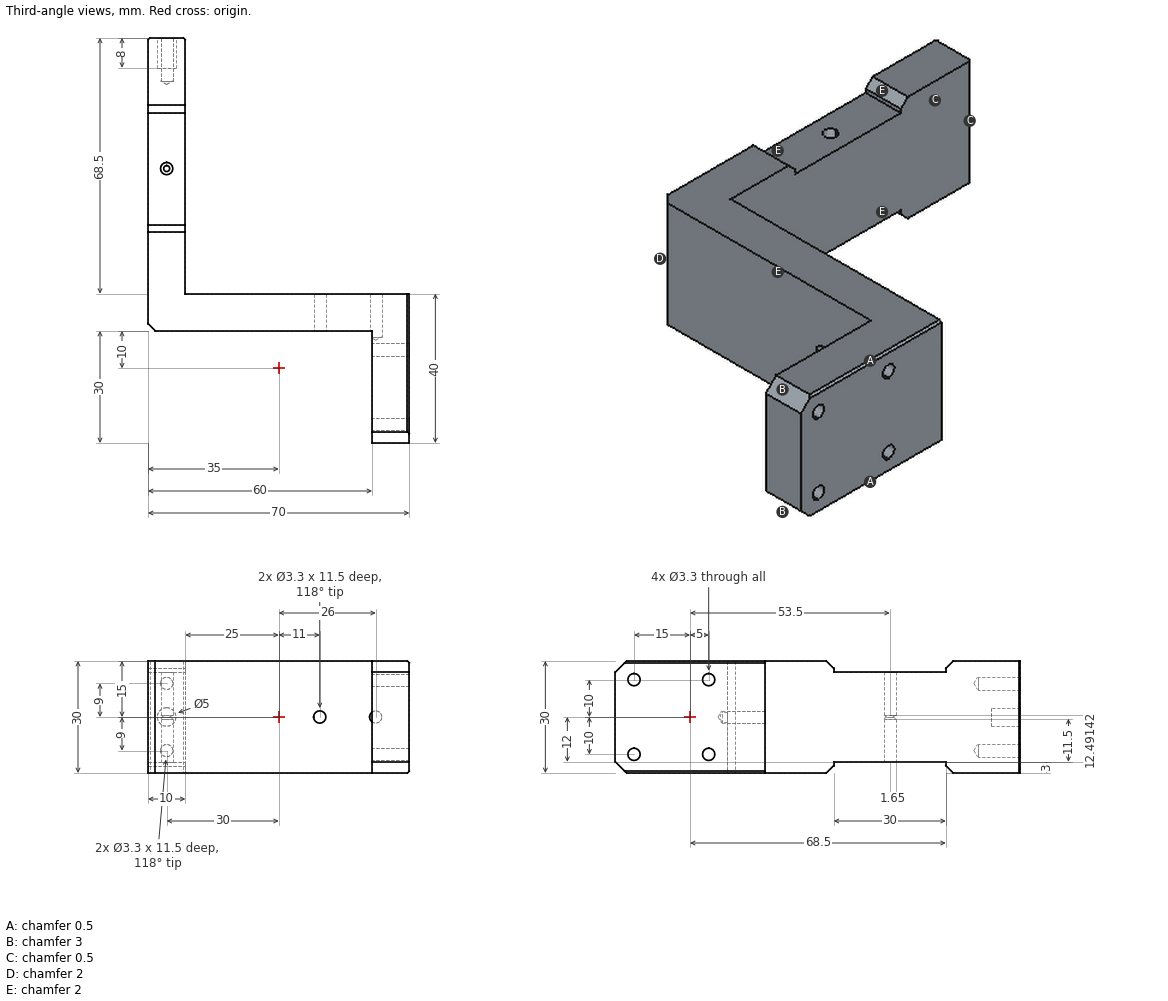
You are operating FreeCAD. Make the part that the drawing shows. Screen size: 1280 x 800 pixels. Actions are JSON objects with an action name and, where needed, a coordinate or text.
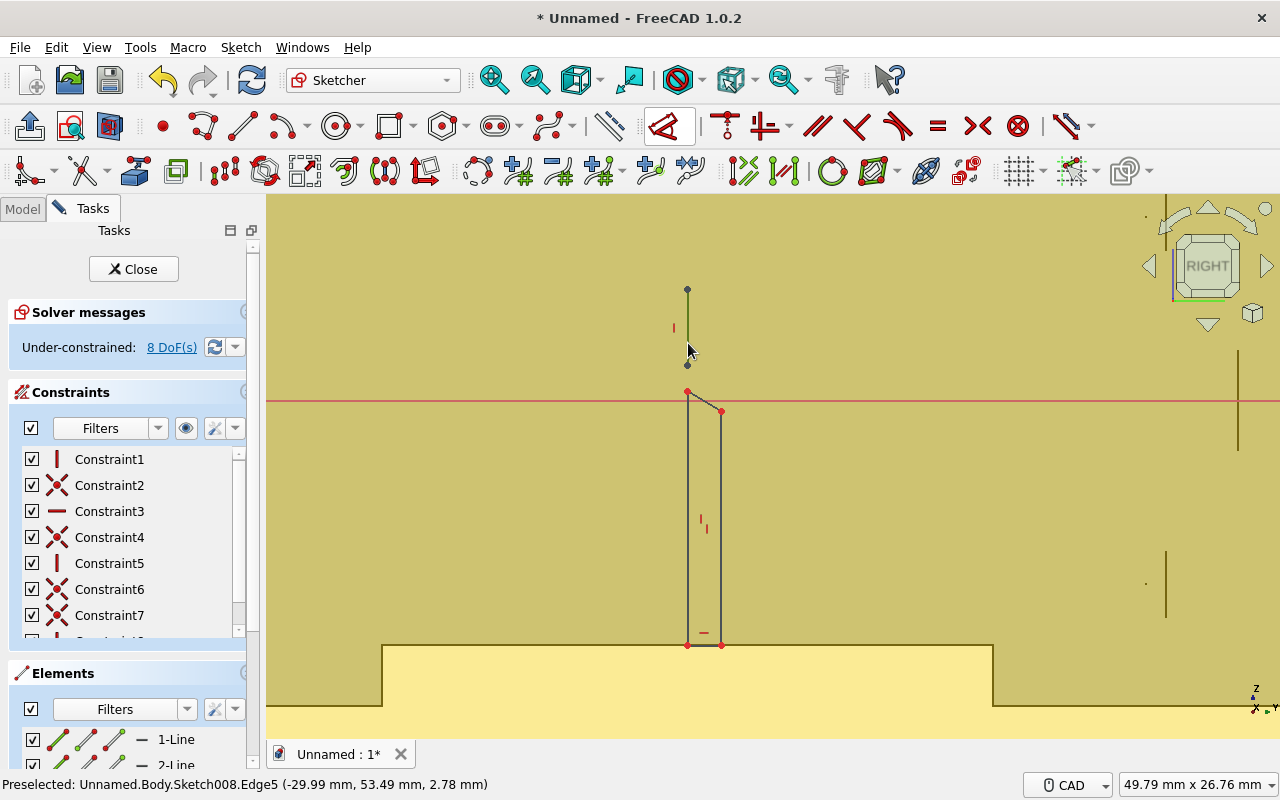
{"action": "left_click", "coordinate": [610, 126]}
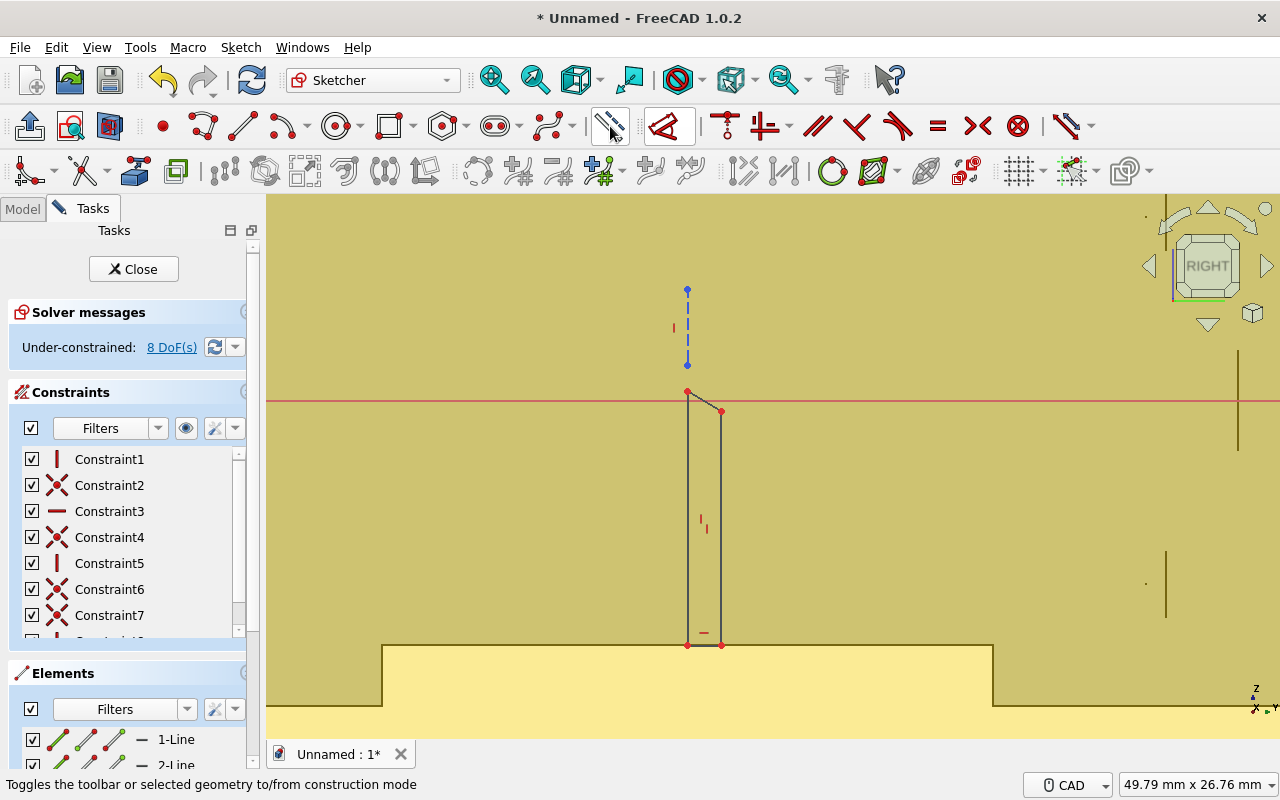
{"action": "left_click", "coordinate": [688, 646]}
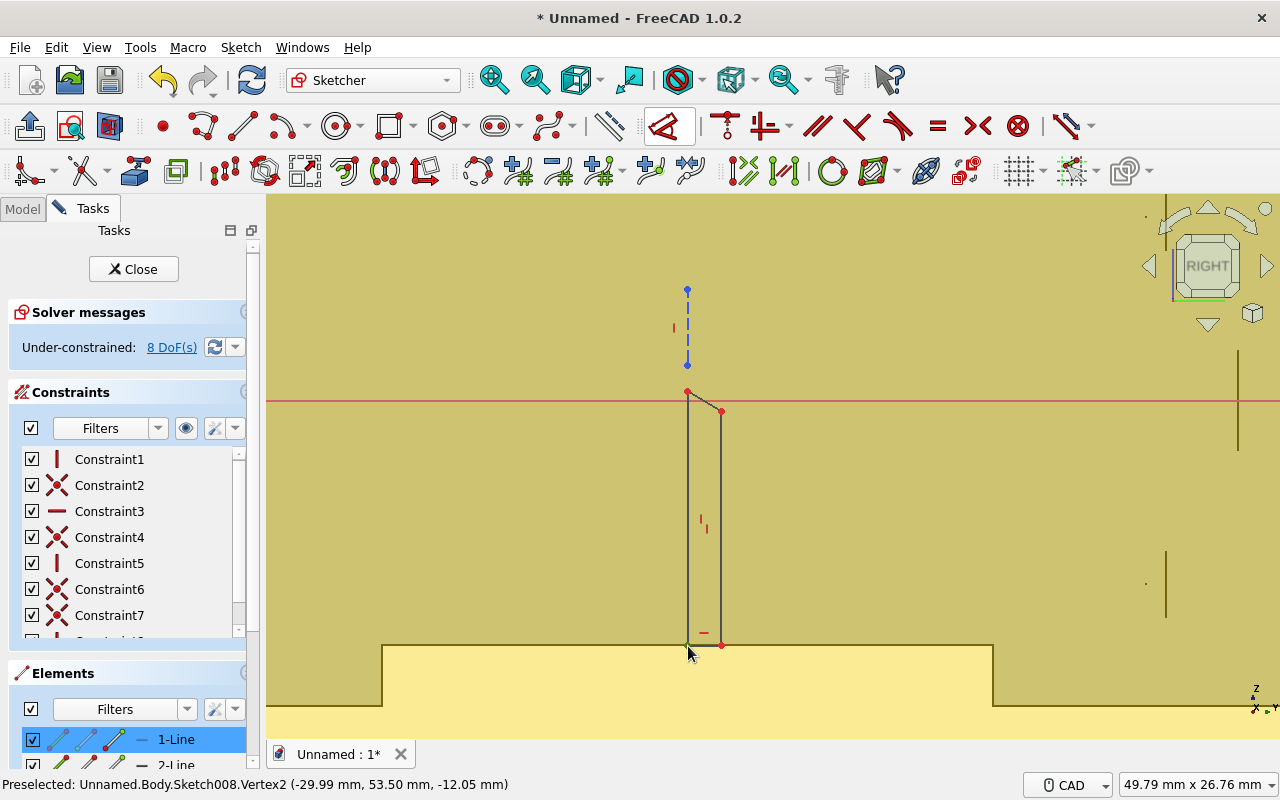
{"action": "key", "text": "i"}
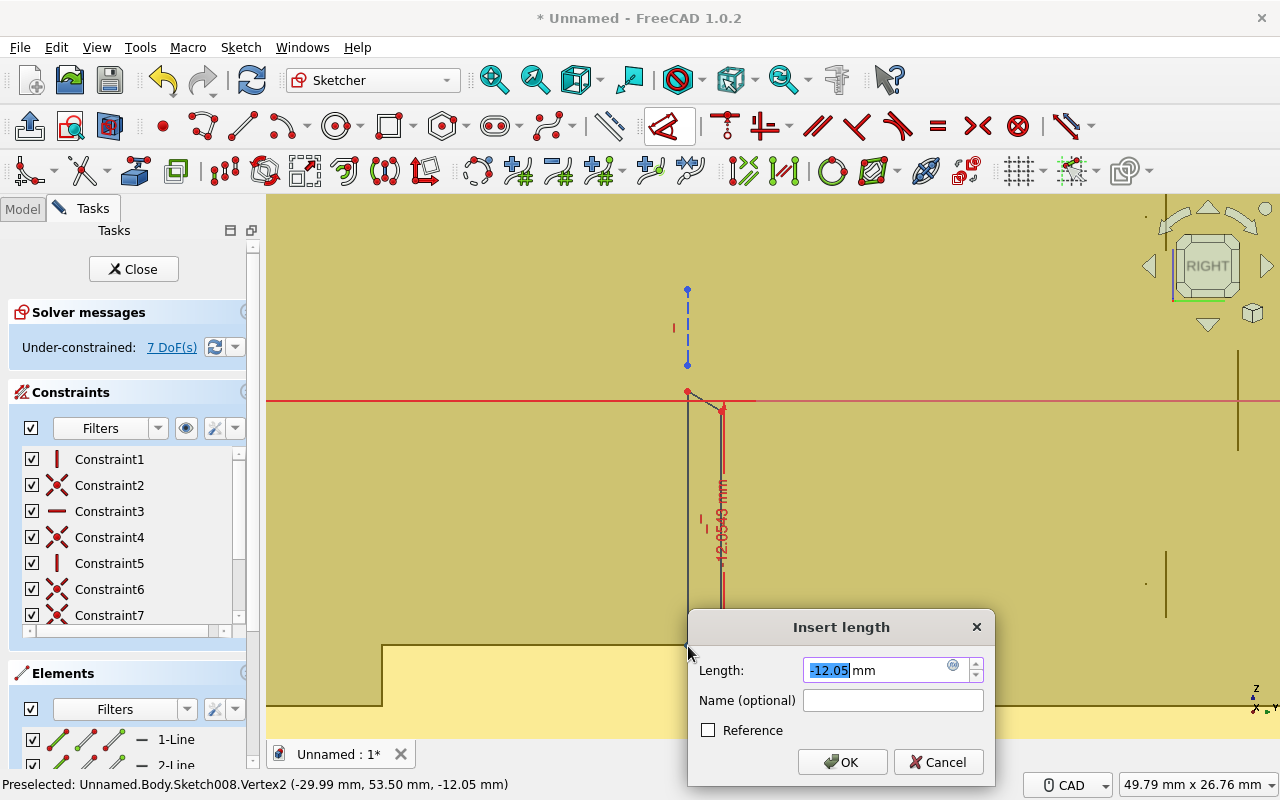
{"action": "type", "text": "-12"}
{"action": "key", "text": "Return"}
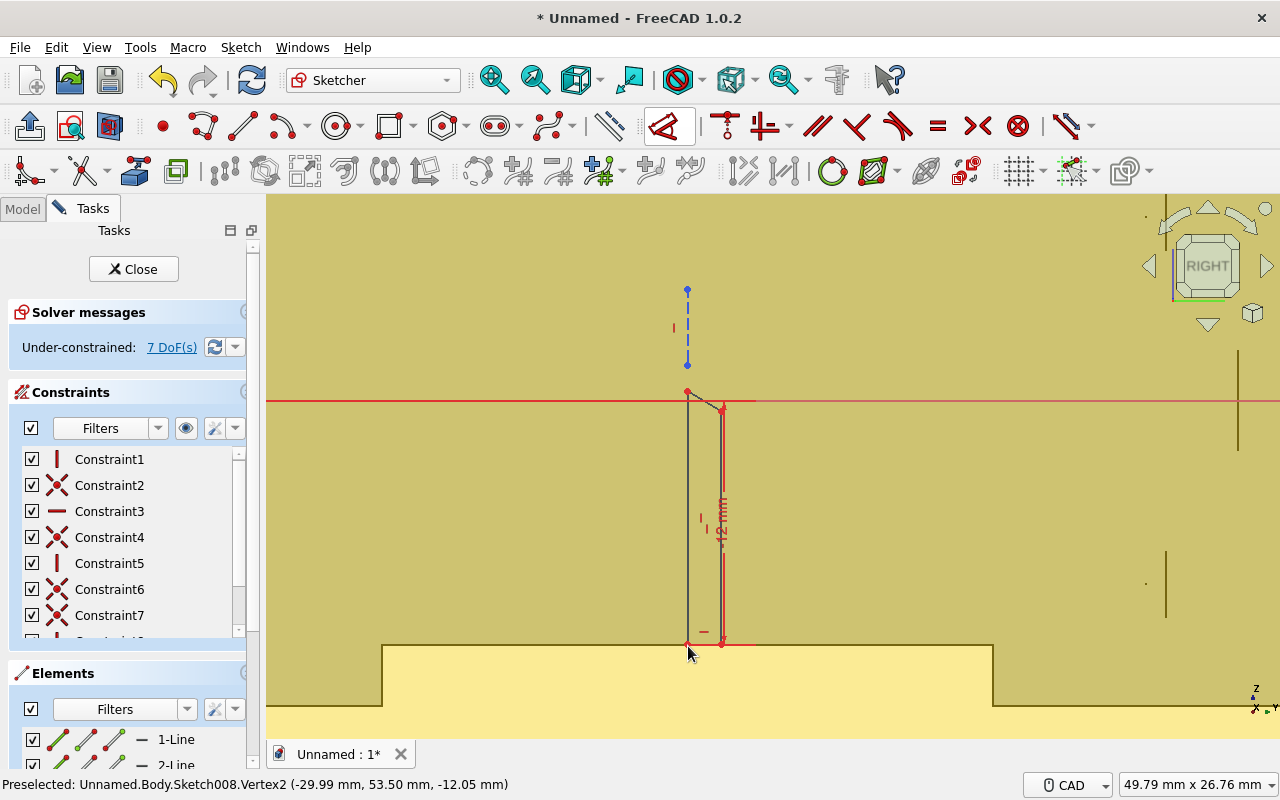
{"action": "scroll", "coordinate": [698, 645], "scroll_direction": "up", "scroll_amount": 2}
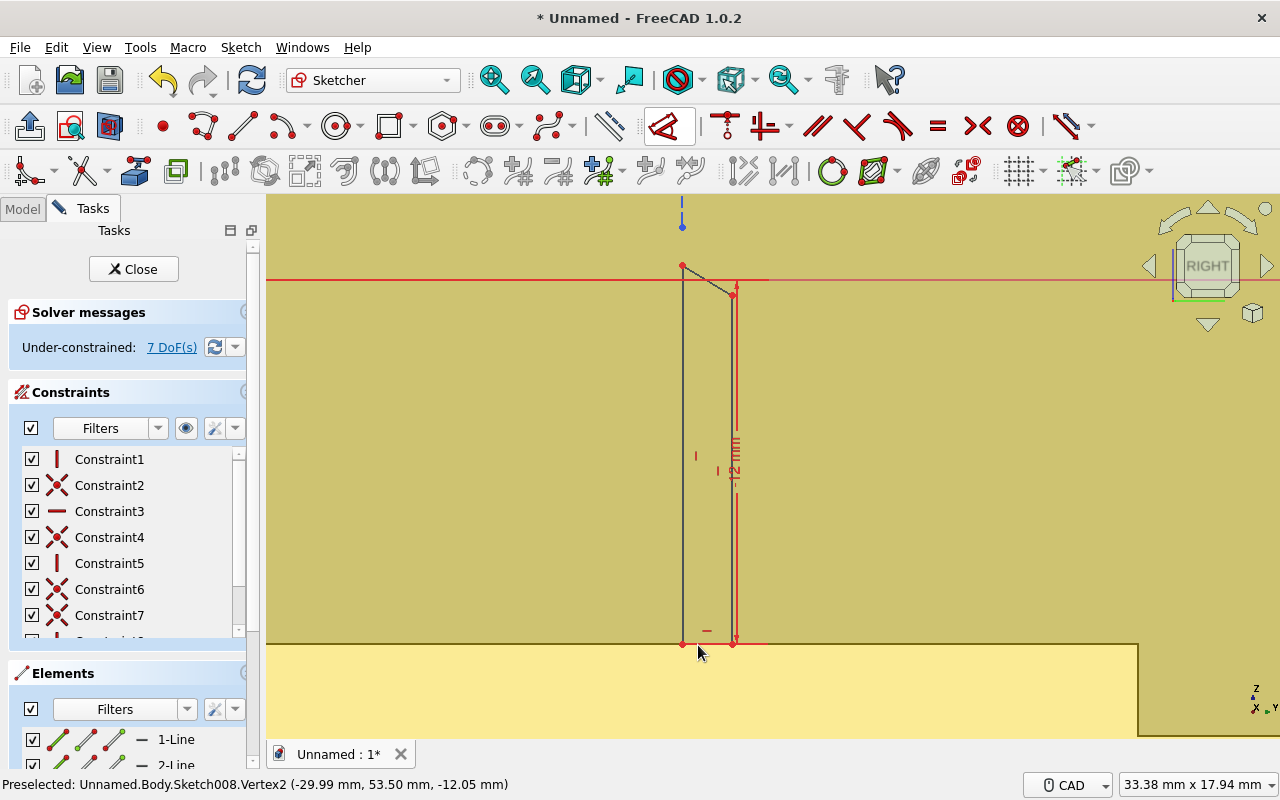
{"action": "left_click", "coordinate": [697, 644]}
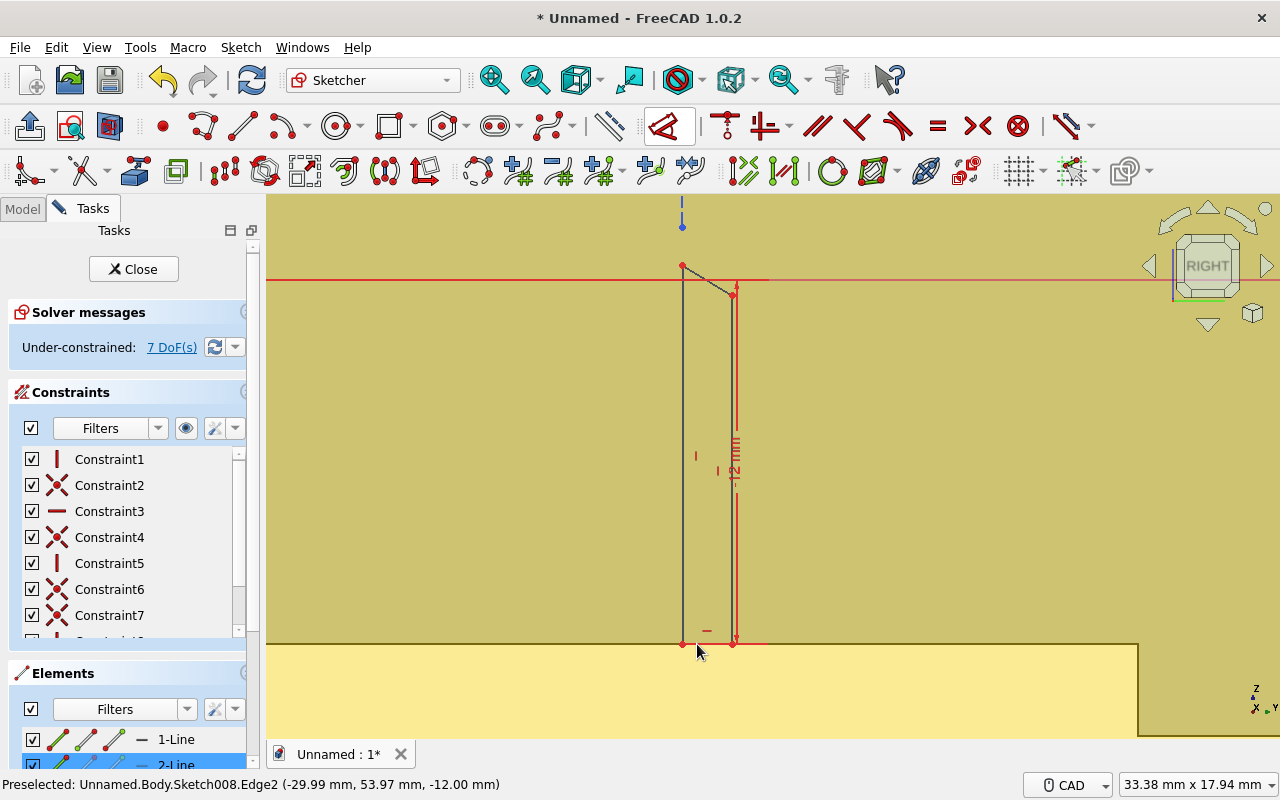
{"action": "left_click", "coordinate": [690, 126]}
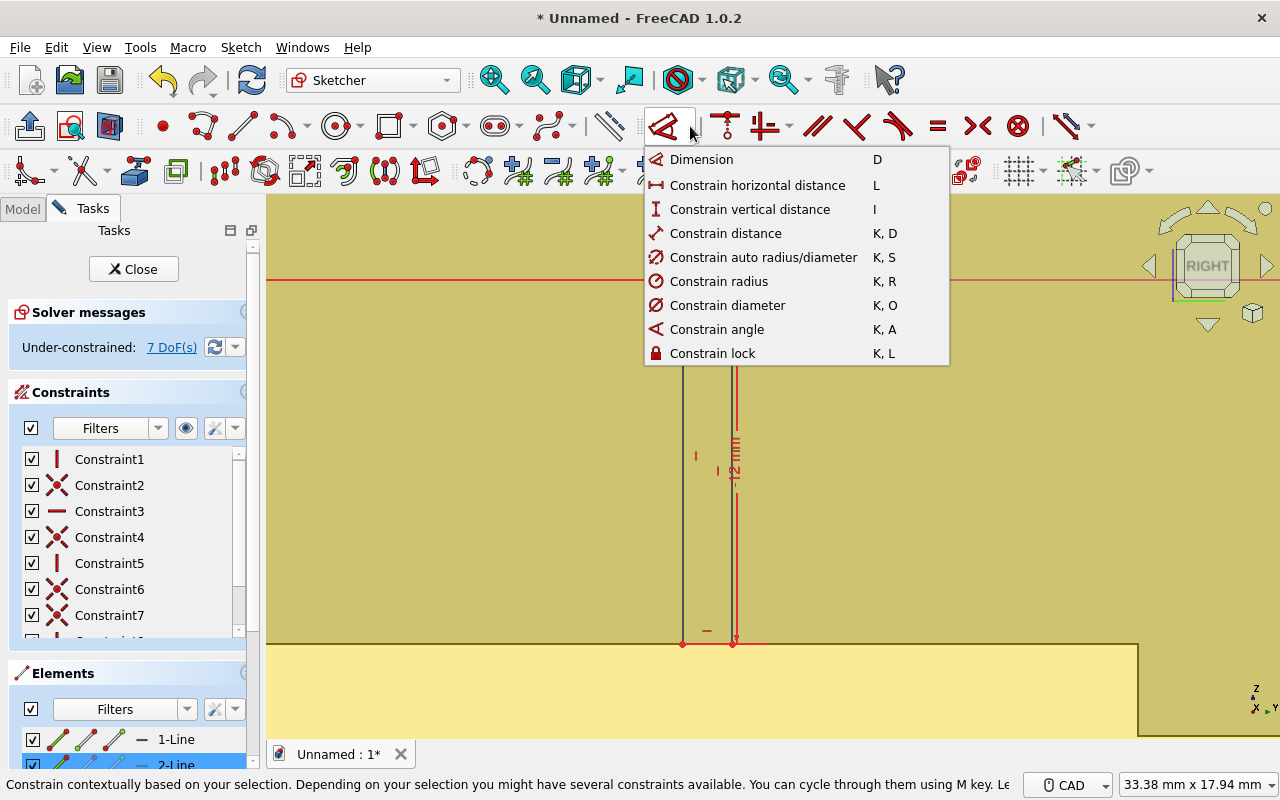
{"action": "left_click", "coordinate": [797, 185]}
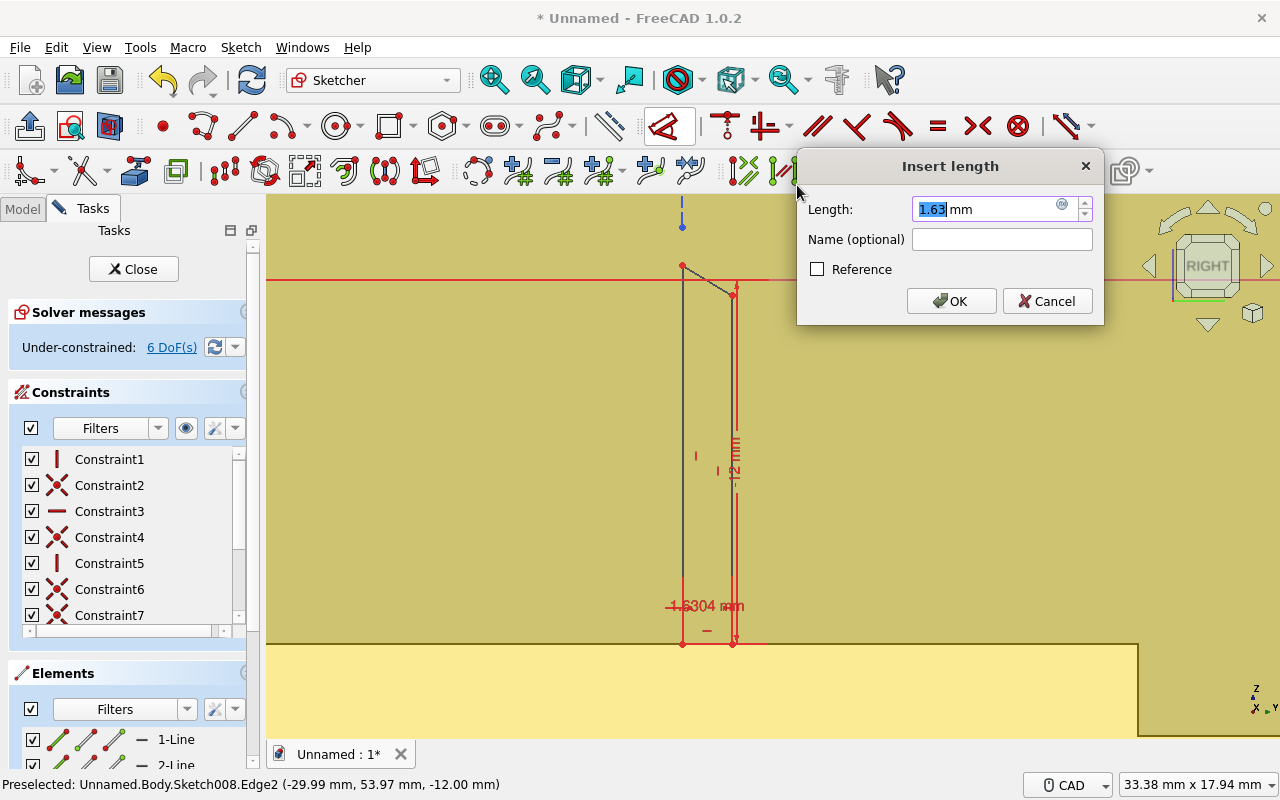
{"action": "type", "text": "1.65"}
{"action": "key", "text": "Return"}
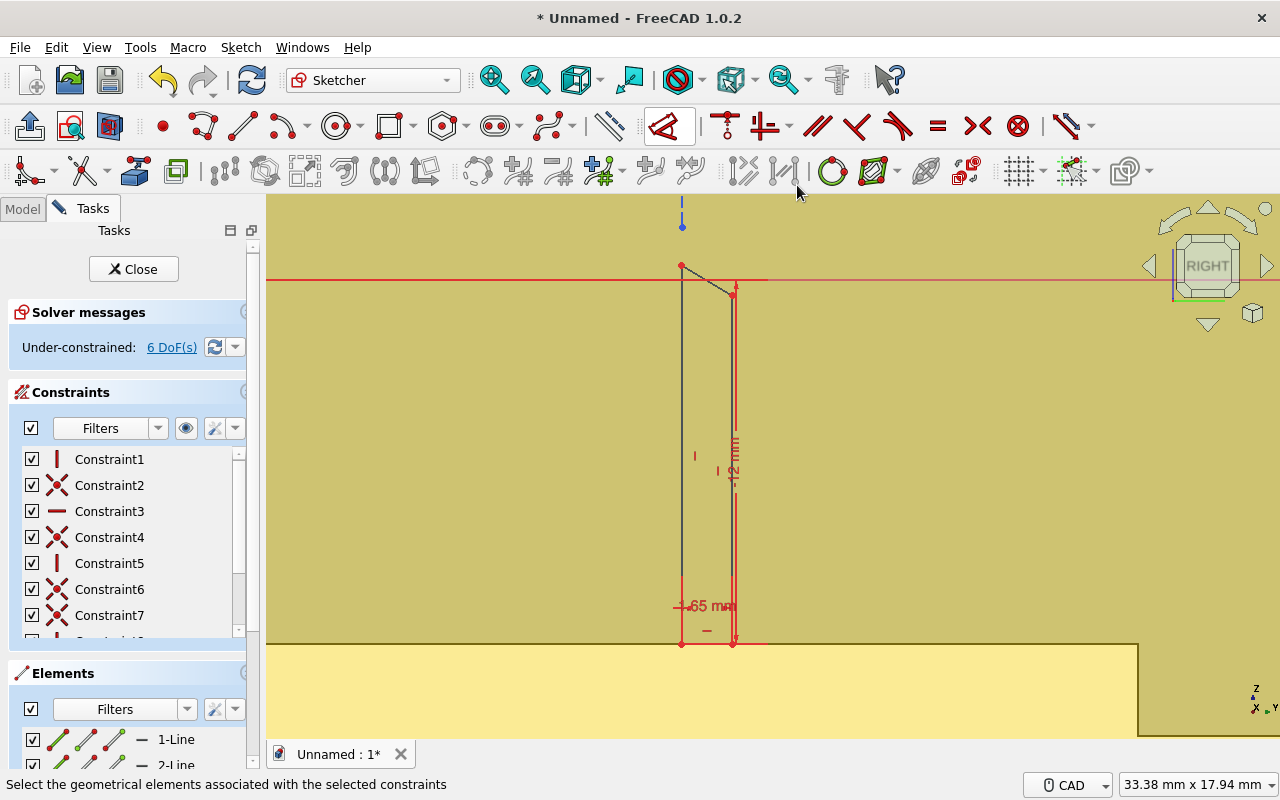
{"action": "left_click", "coordinate": [732, 540]}